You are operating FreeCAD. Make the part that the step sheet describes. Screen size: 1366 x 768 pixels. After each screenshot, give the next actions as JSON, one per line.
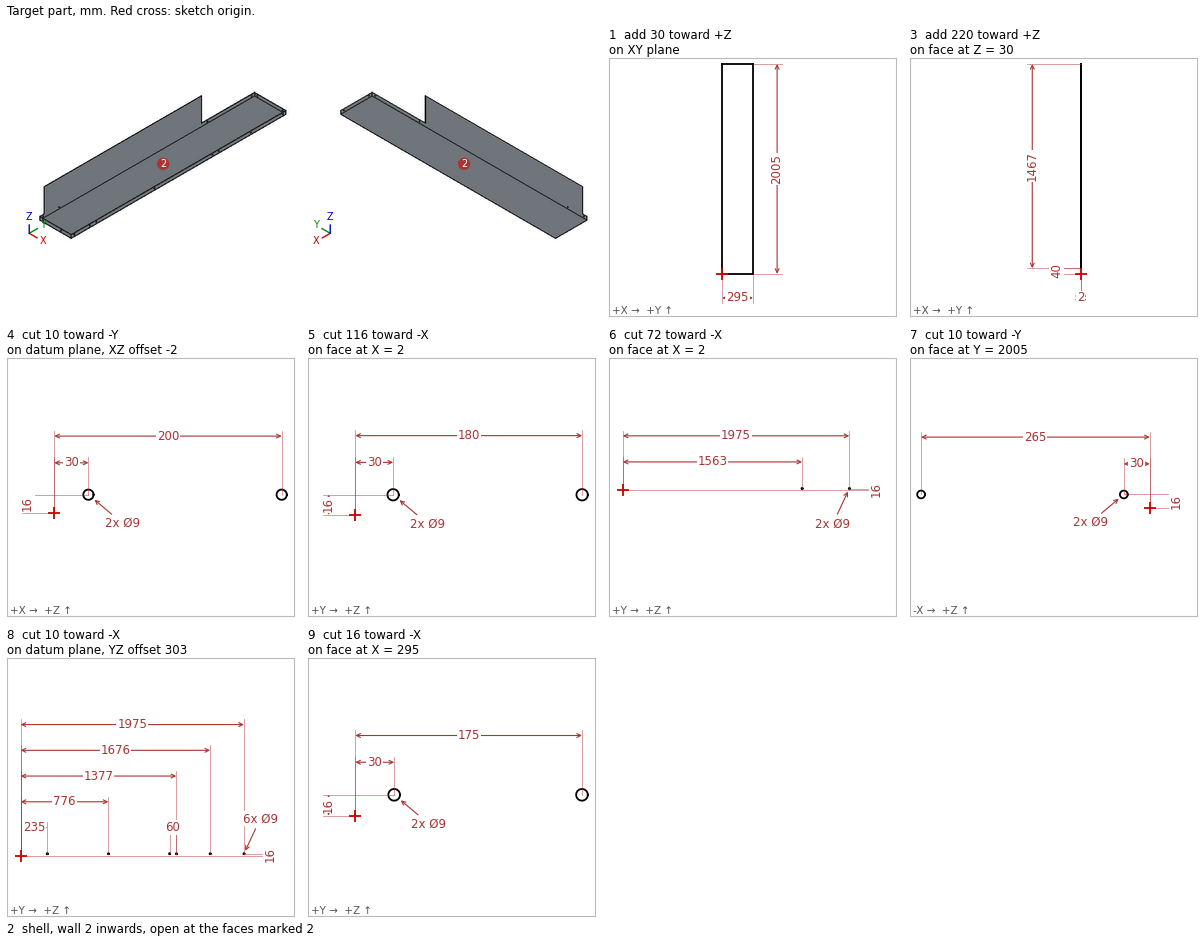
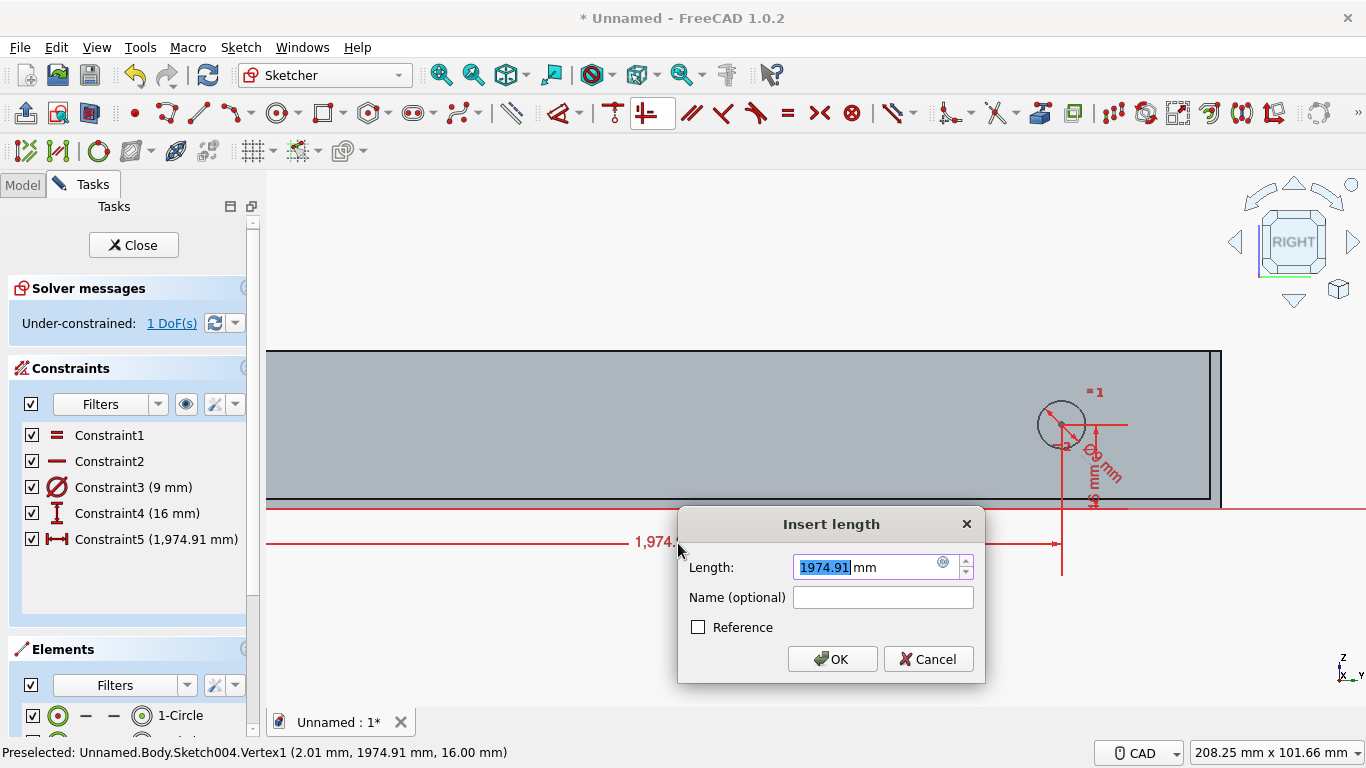
{"action": "type", "text": "1975"}
{"action": "key", "text": "Return"}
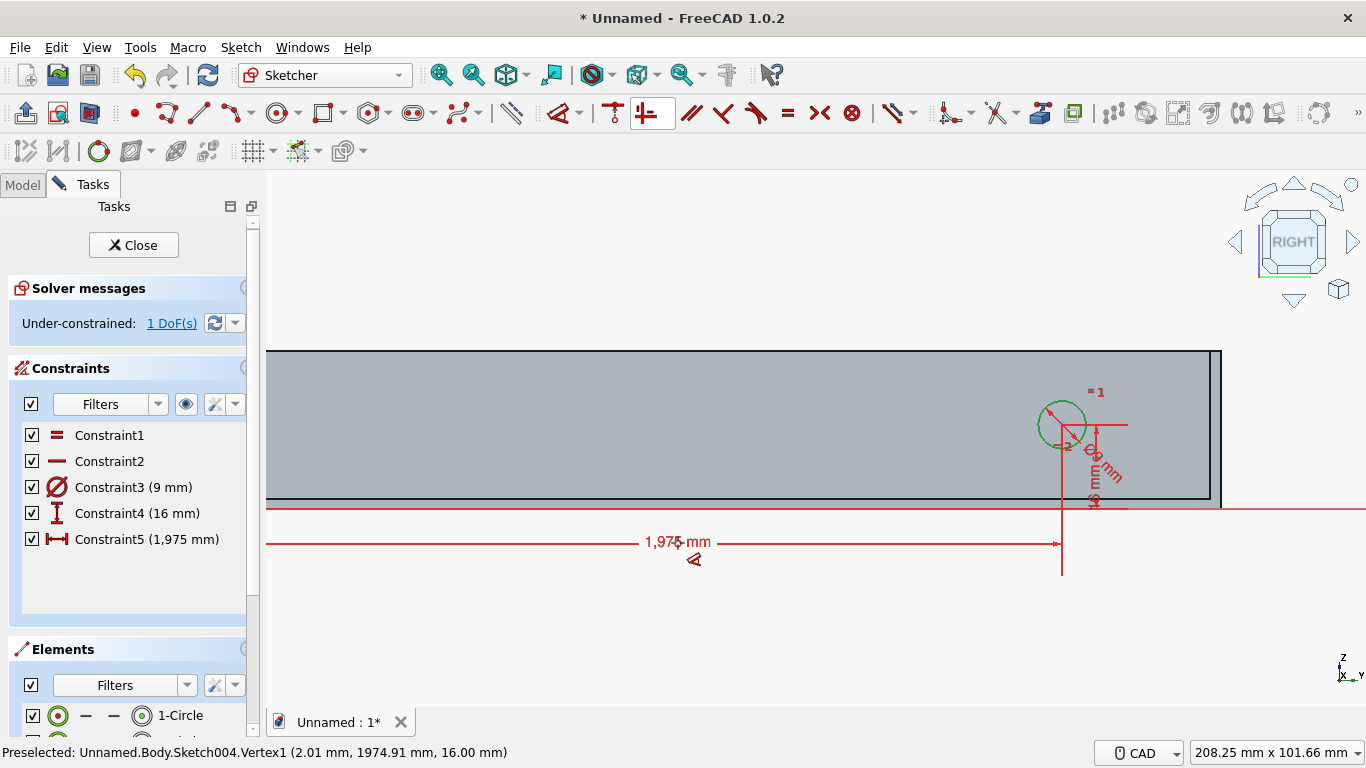
{"action": "scroll", "coordinate": [1081, 444], "scroll_direction": "down", "scroll_amount": 6}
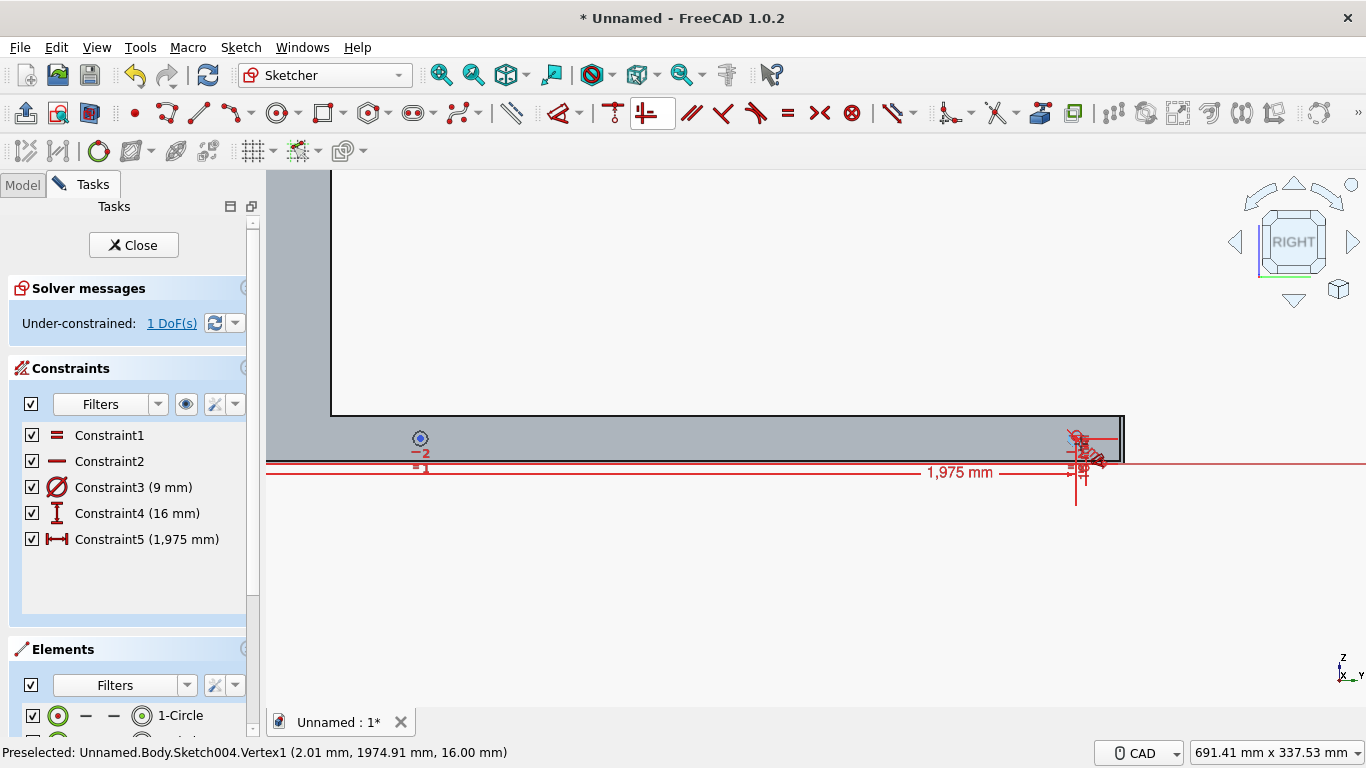
{"action": "left_click", "coordinate": [420, 439]}
{"action": "left_click", "coordinate": [357, 498]}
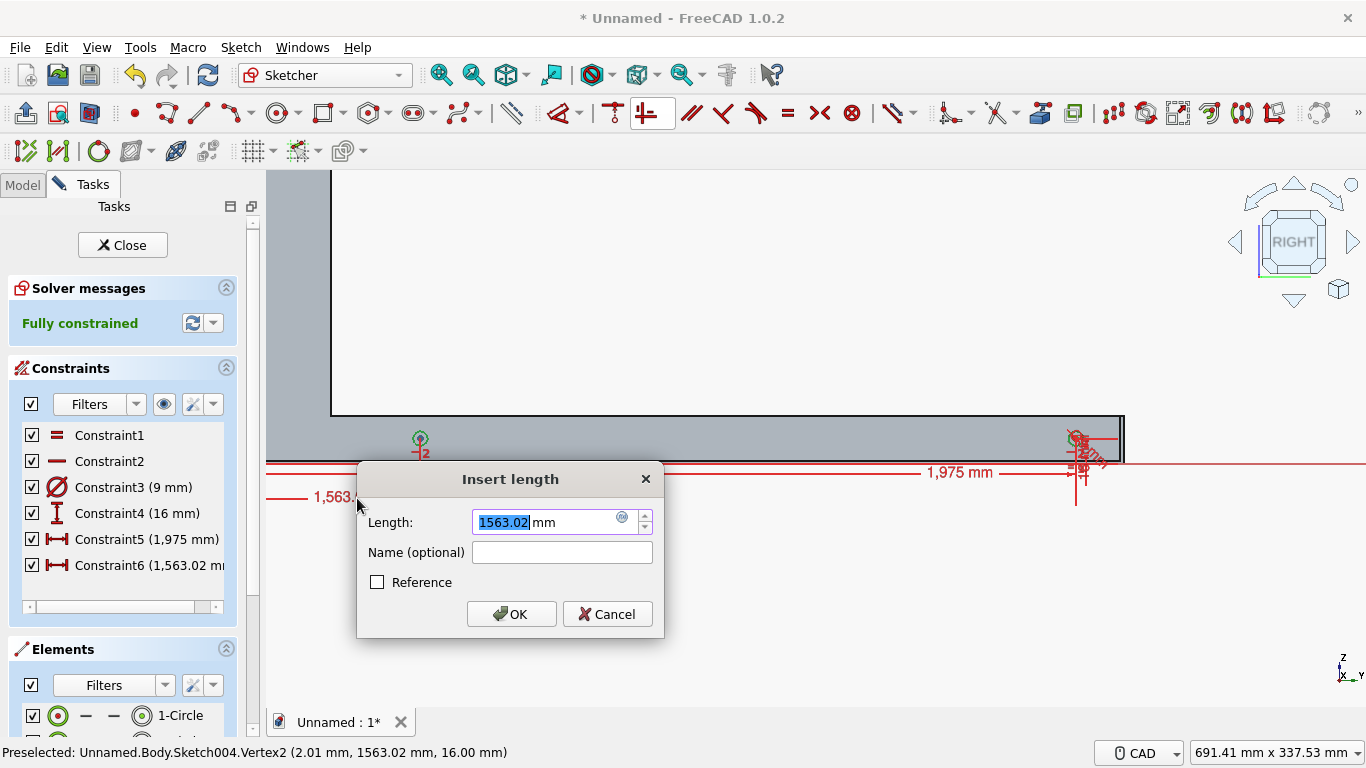
{"action": "type", "text": "1563"}
{"action": "key", "text": "Return"}
{"action": "key", "text": "Escape"}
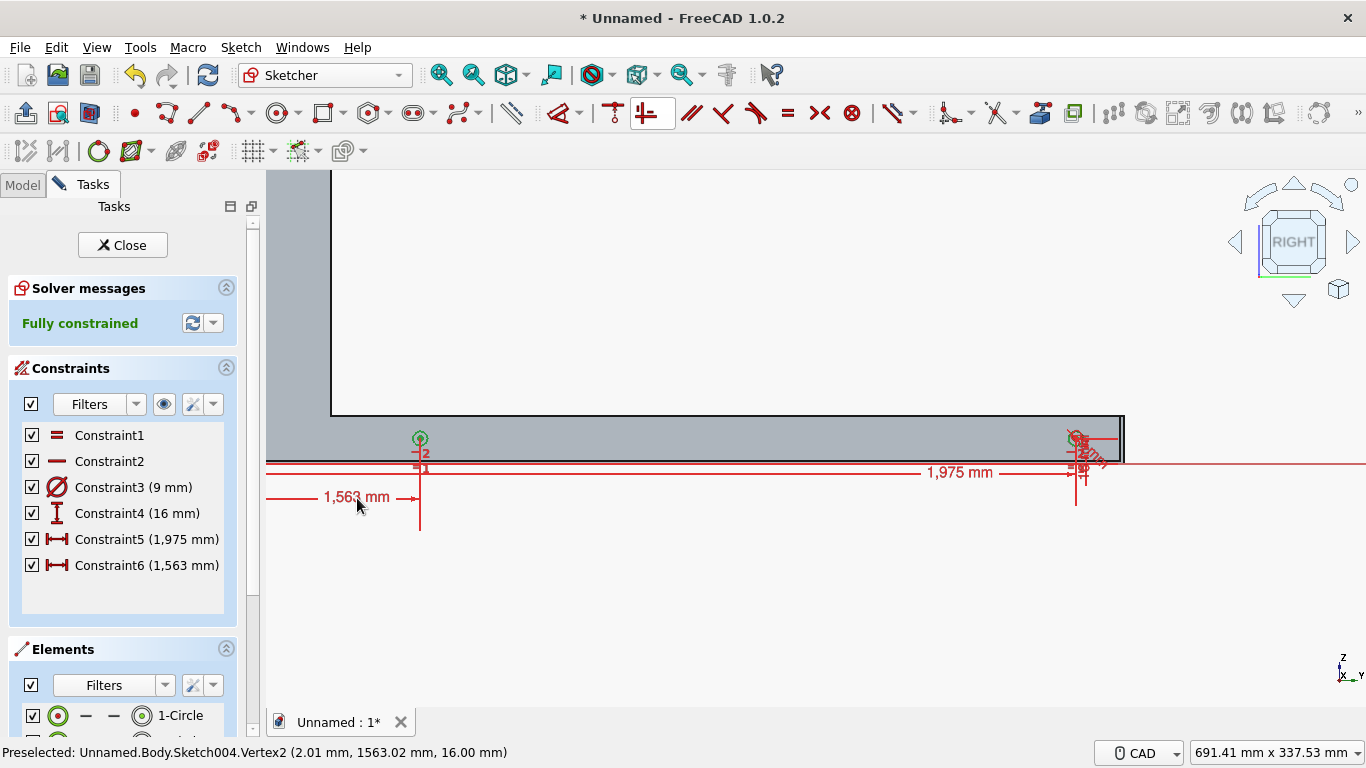
{"action": "left_click", "coordinate": [123, 245]}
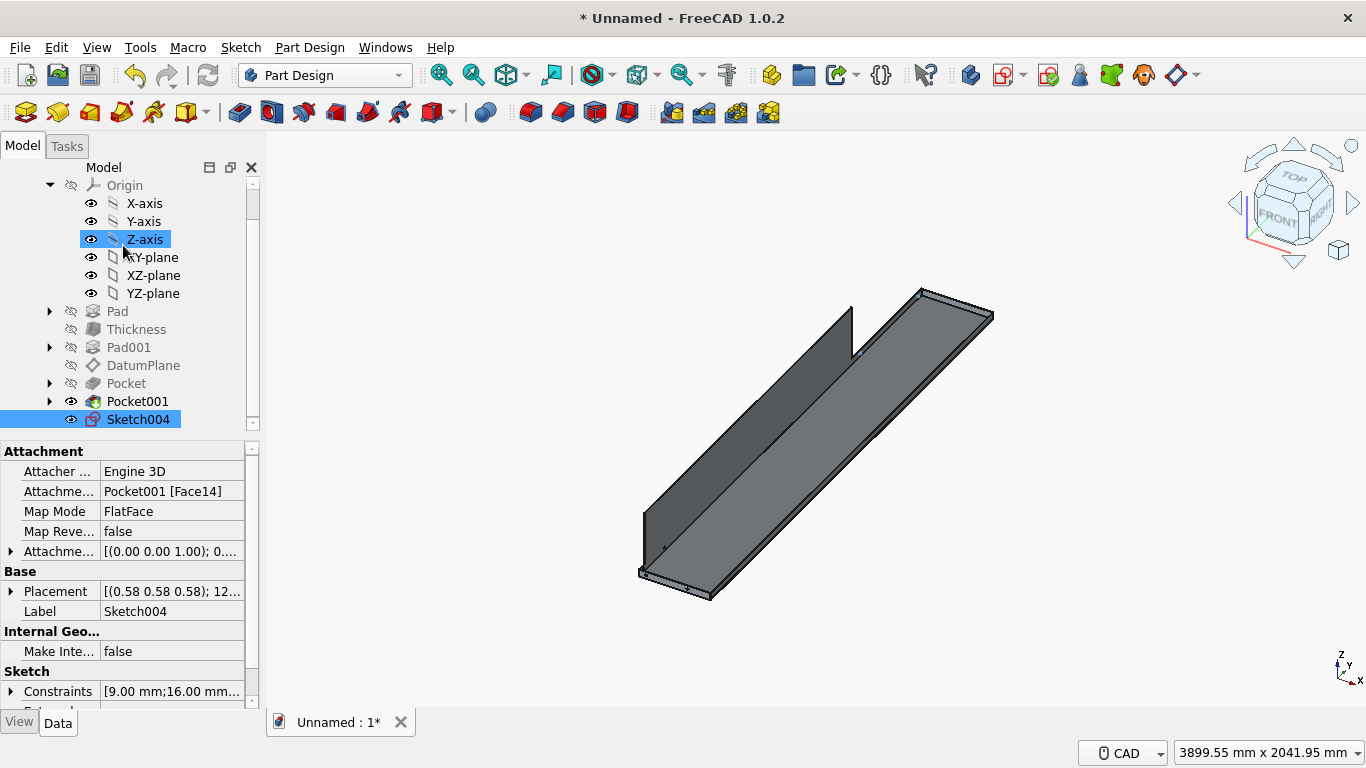
{"action": "left_click", "coordinate": [240, 112]}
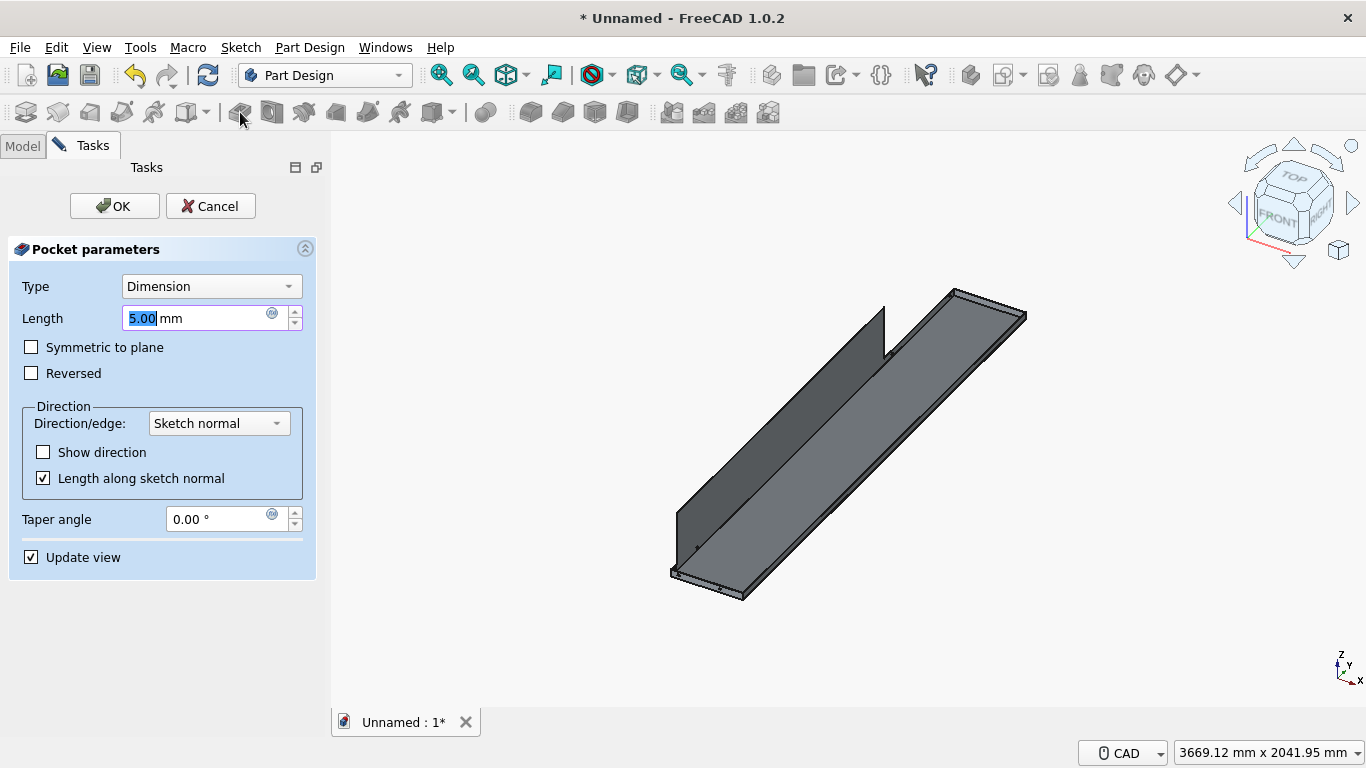
{"action": "type", "text": "72"}
{"action": "key", "text": "Tab"}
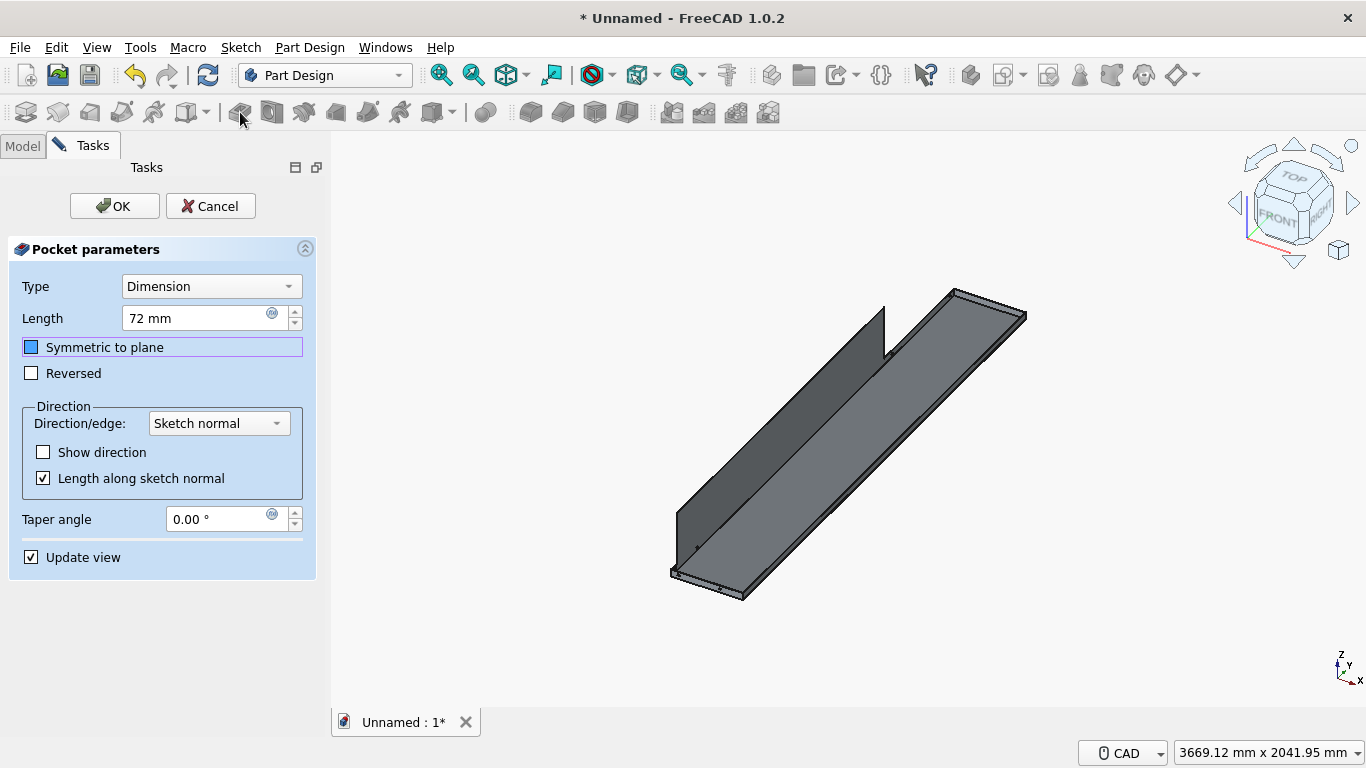
{"action": "left_click", "coordinate": [115, 206]}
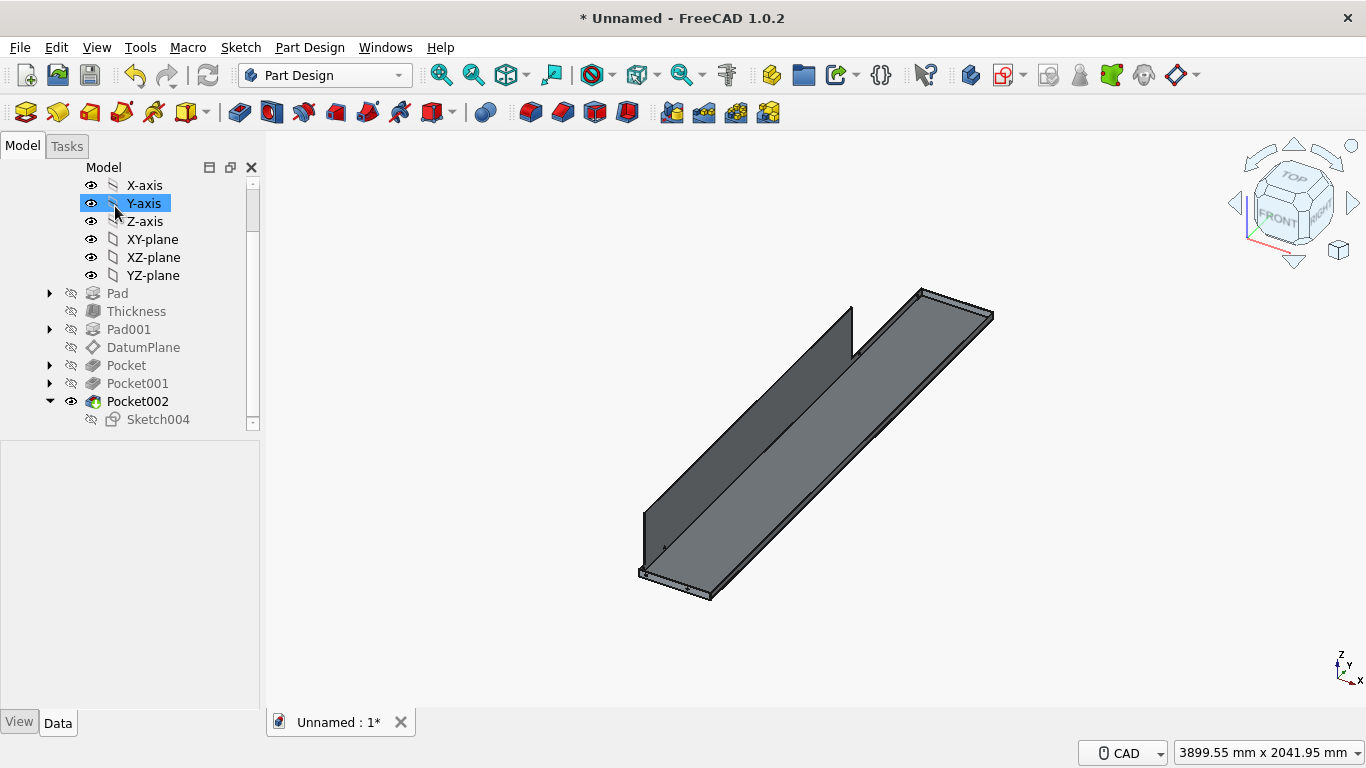
{"action": "key", "text": "4"}